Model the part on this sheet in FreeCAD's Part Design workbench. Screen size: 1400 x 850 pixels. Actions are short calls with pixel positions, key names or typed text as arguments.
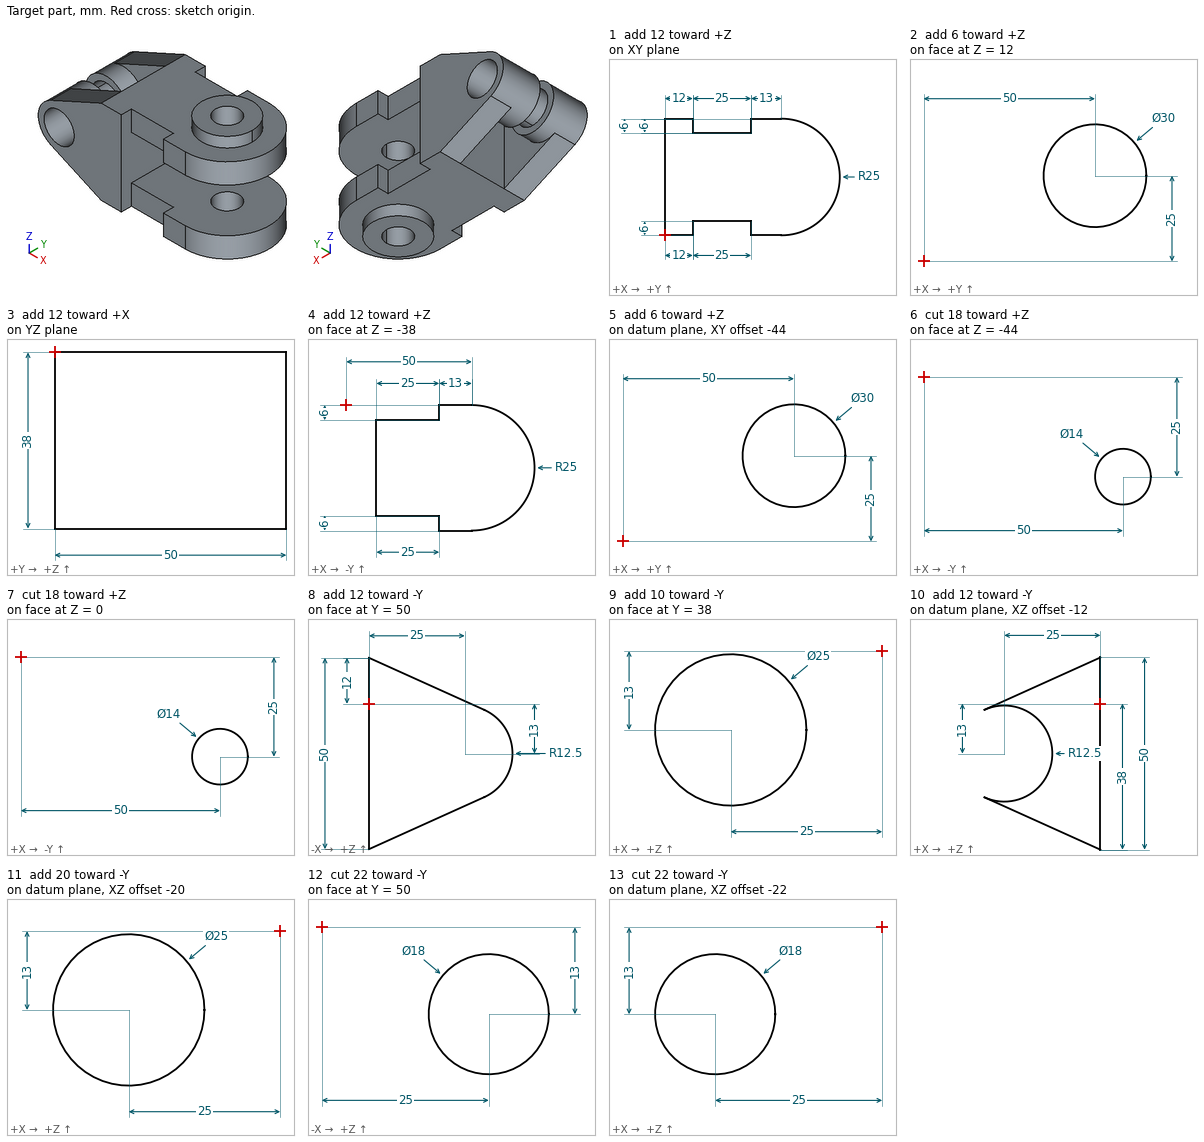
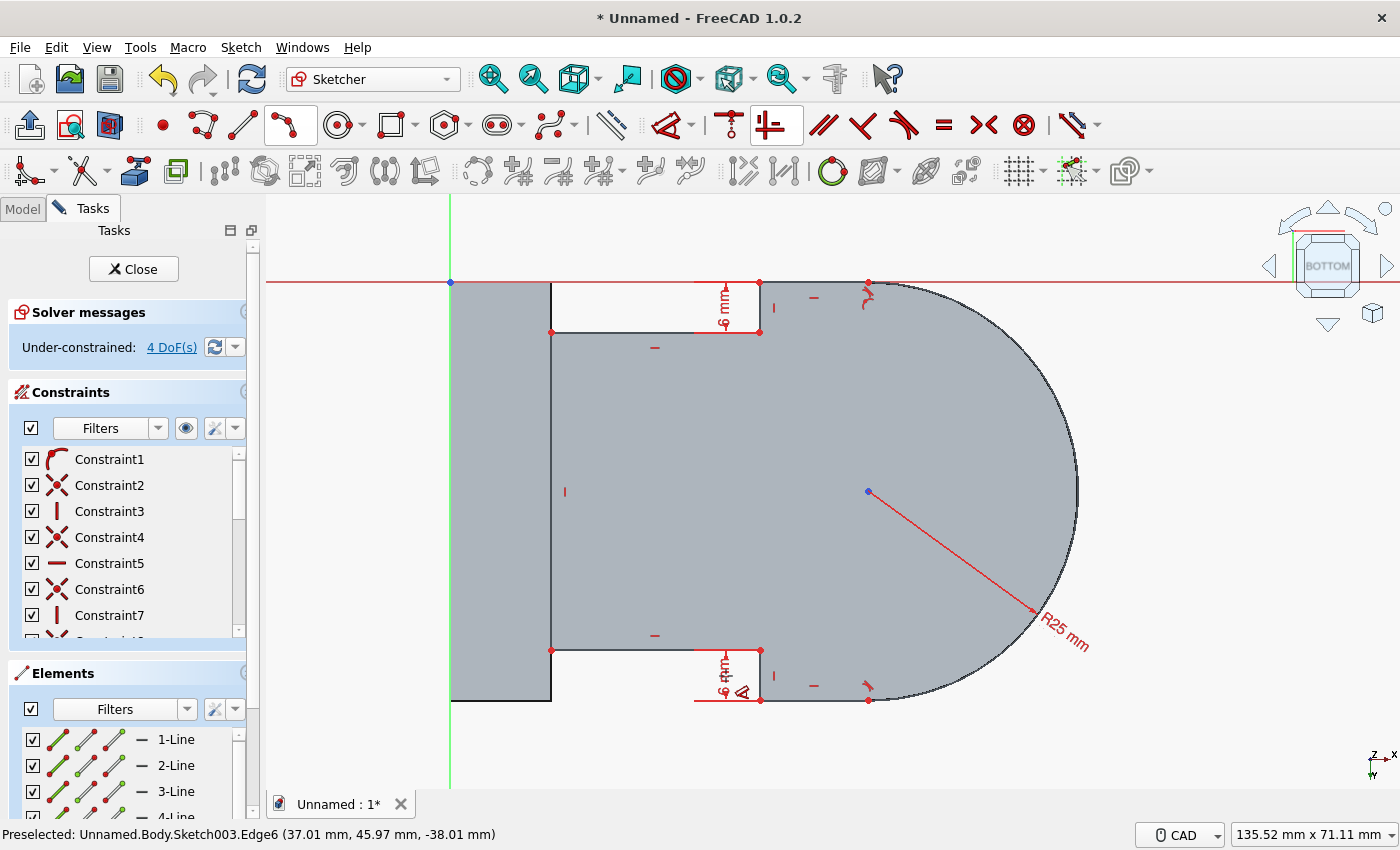
click(836, 282)
click(814, 248)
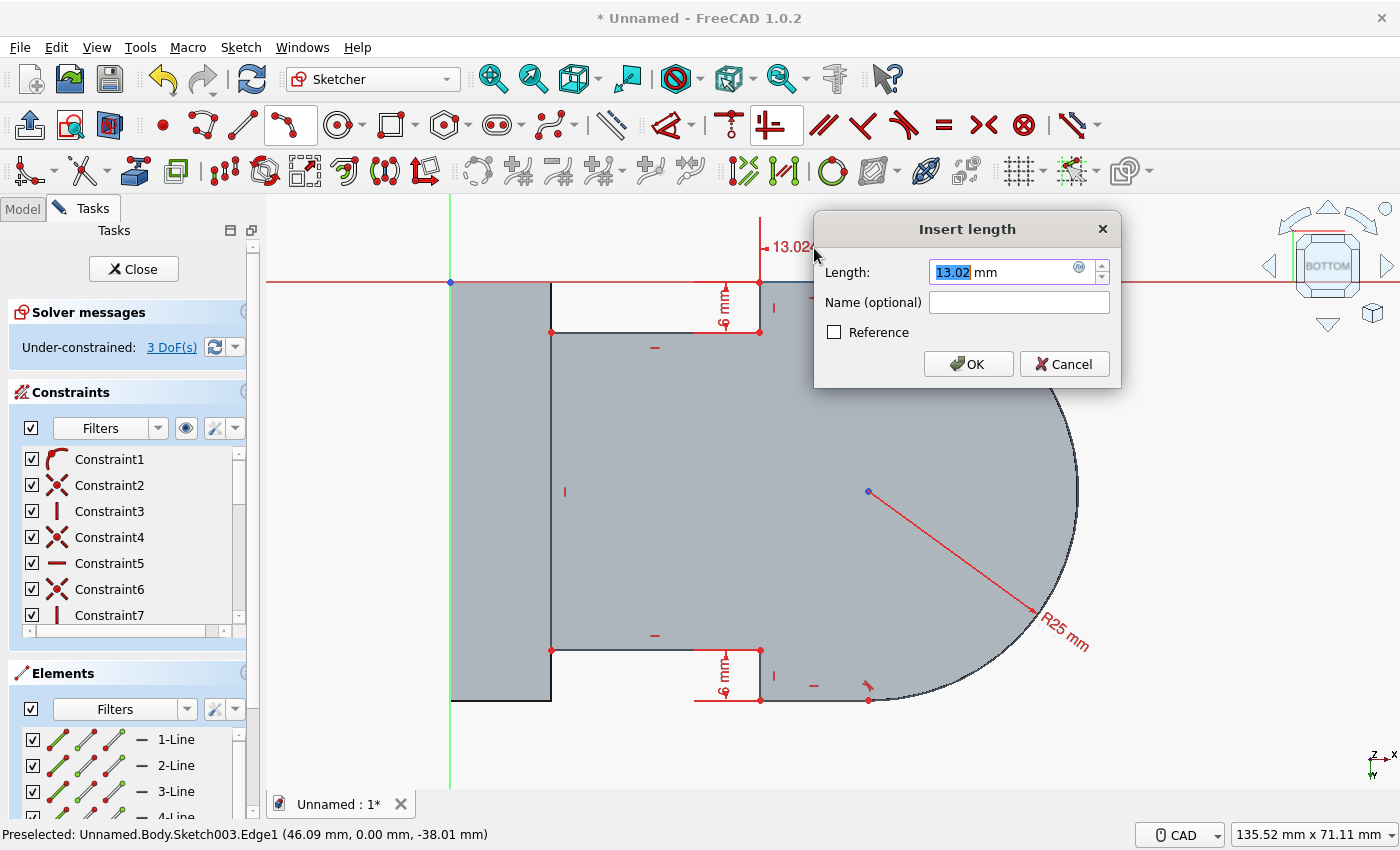
text(13)
key(Return)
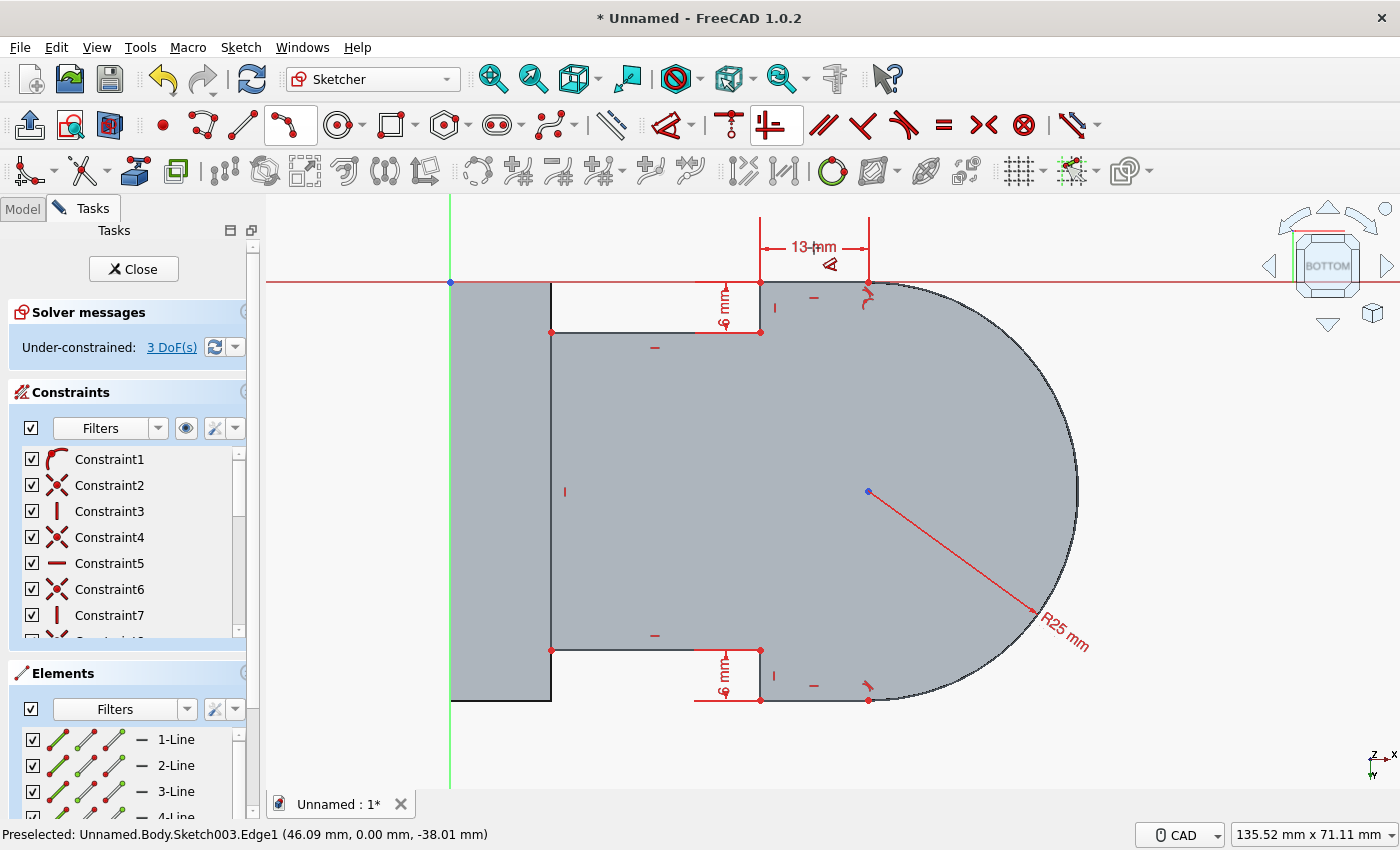
click(697, 333)
click(656, 299)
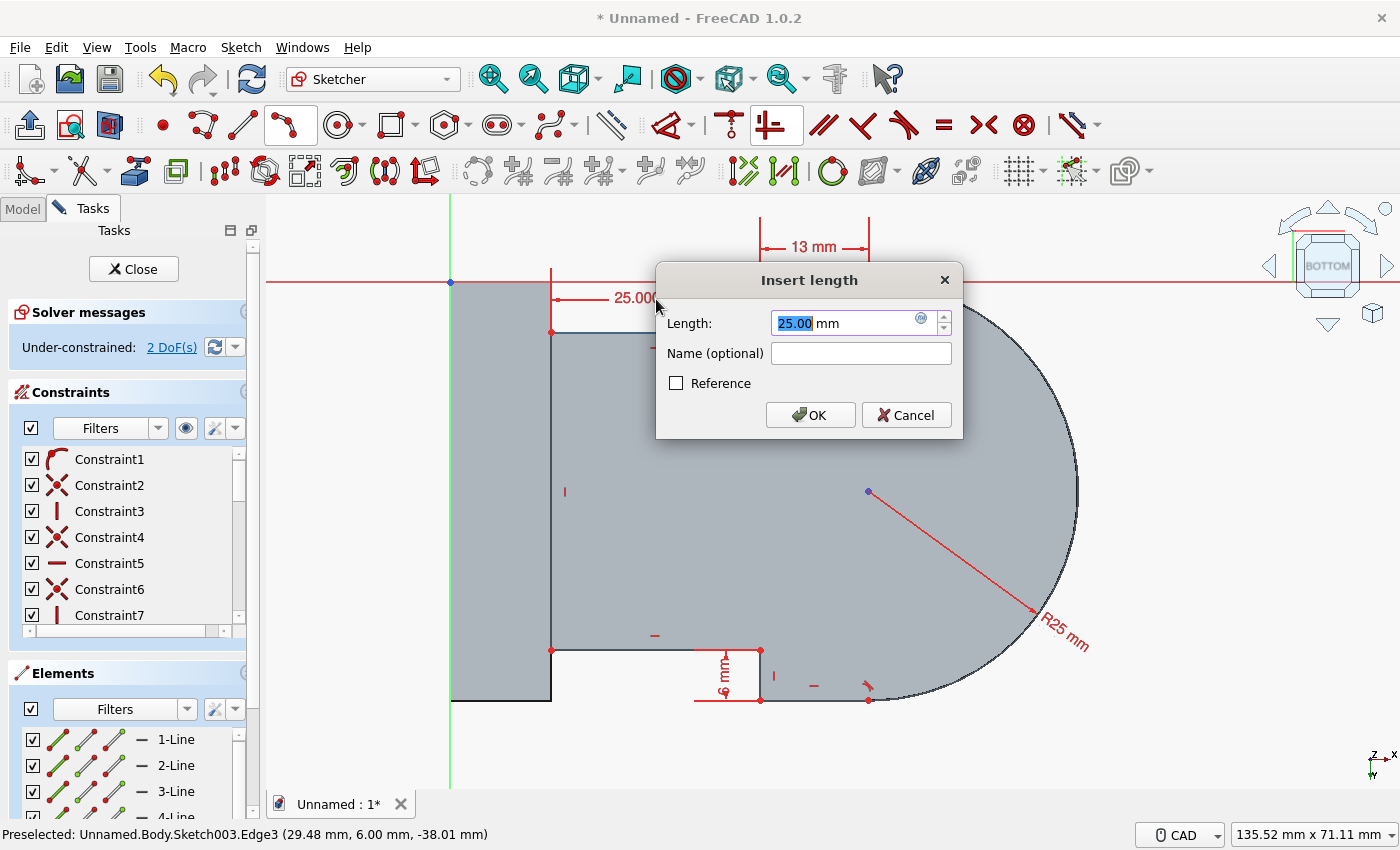
text(25)
key(Return)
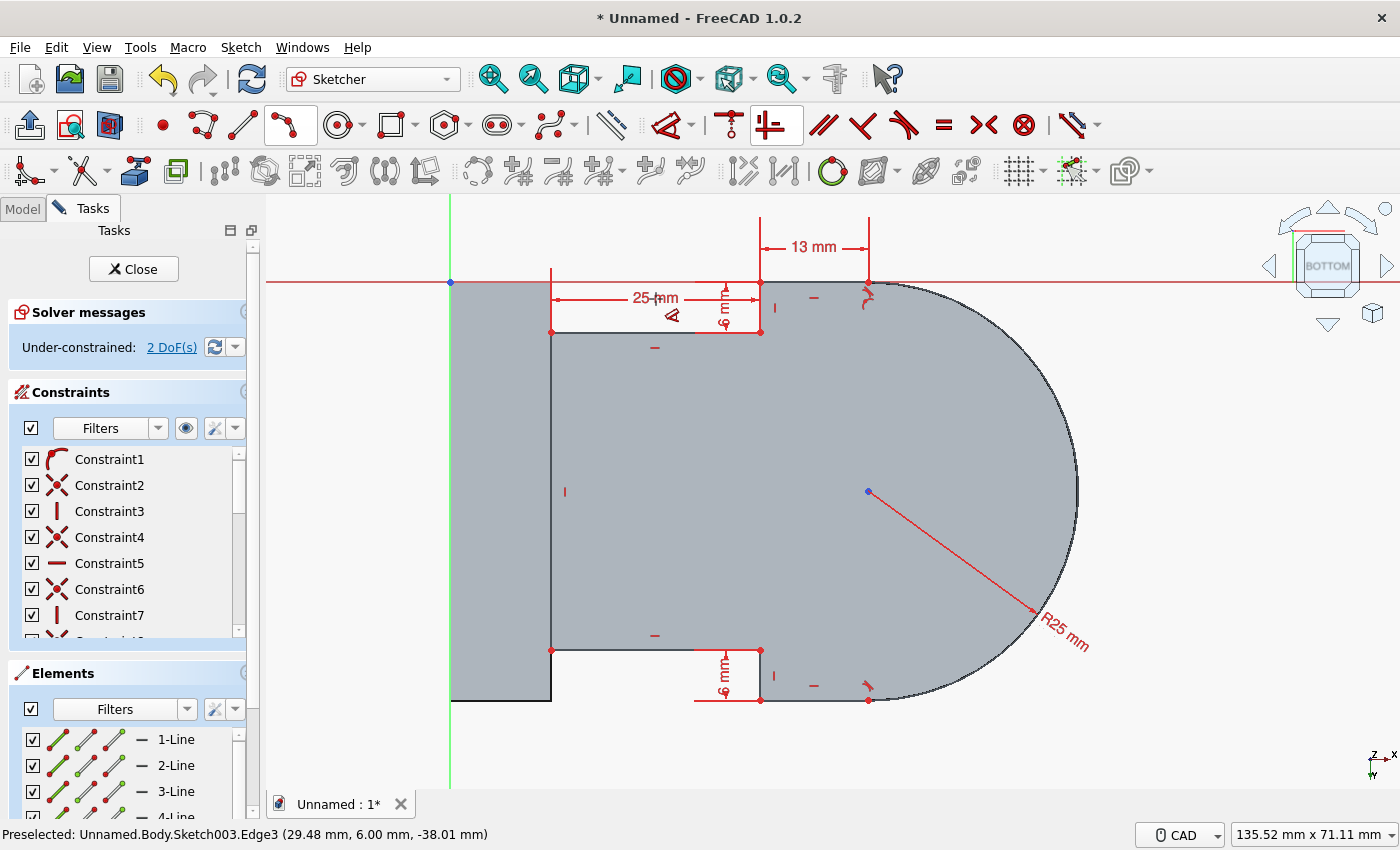
click(614, 650)
click(656, 684)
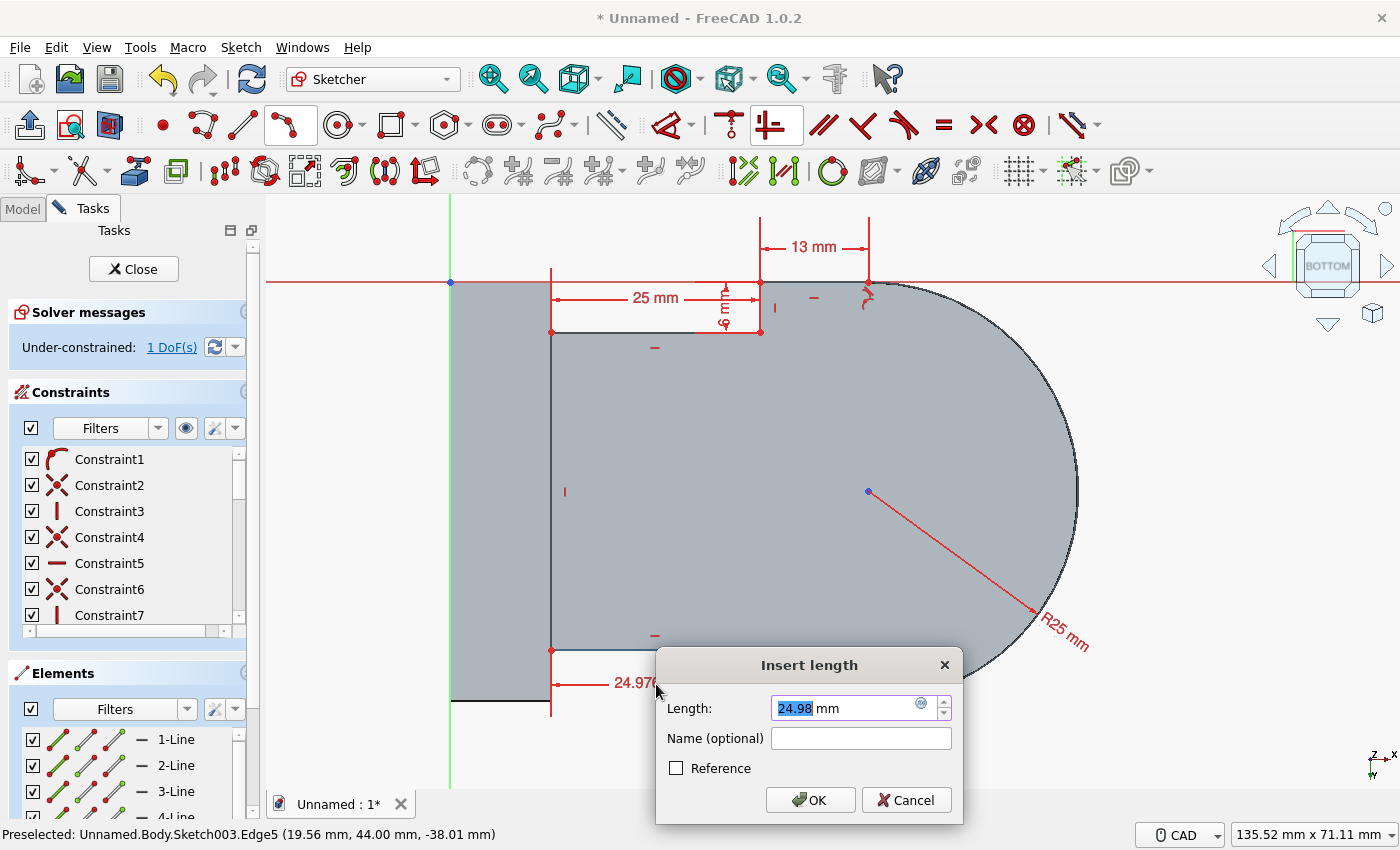
text(25)
key(Return)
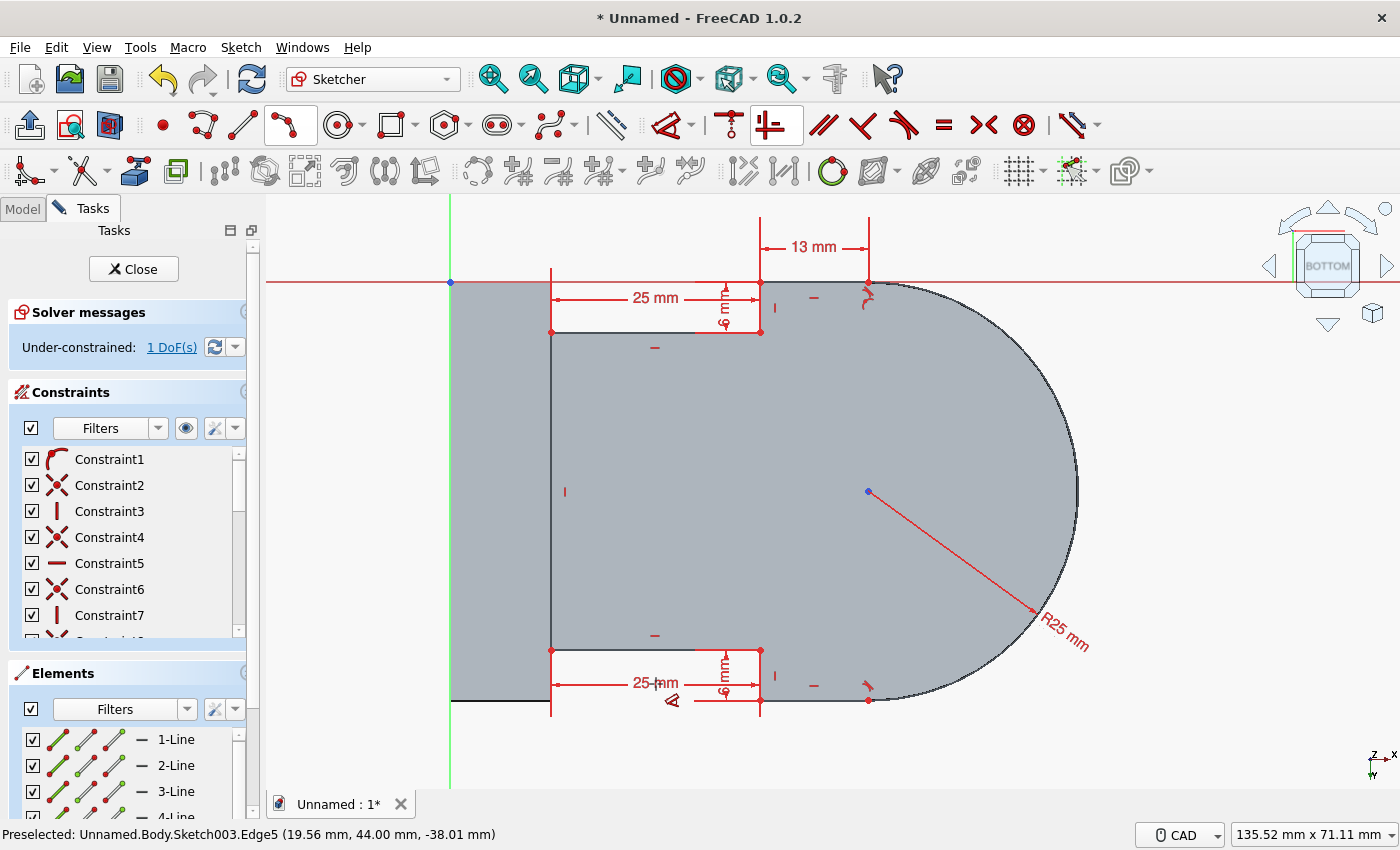
click(869, 282)
click(660, 248)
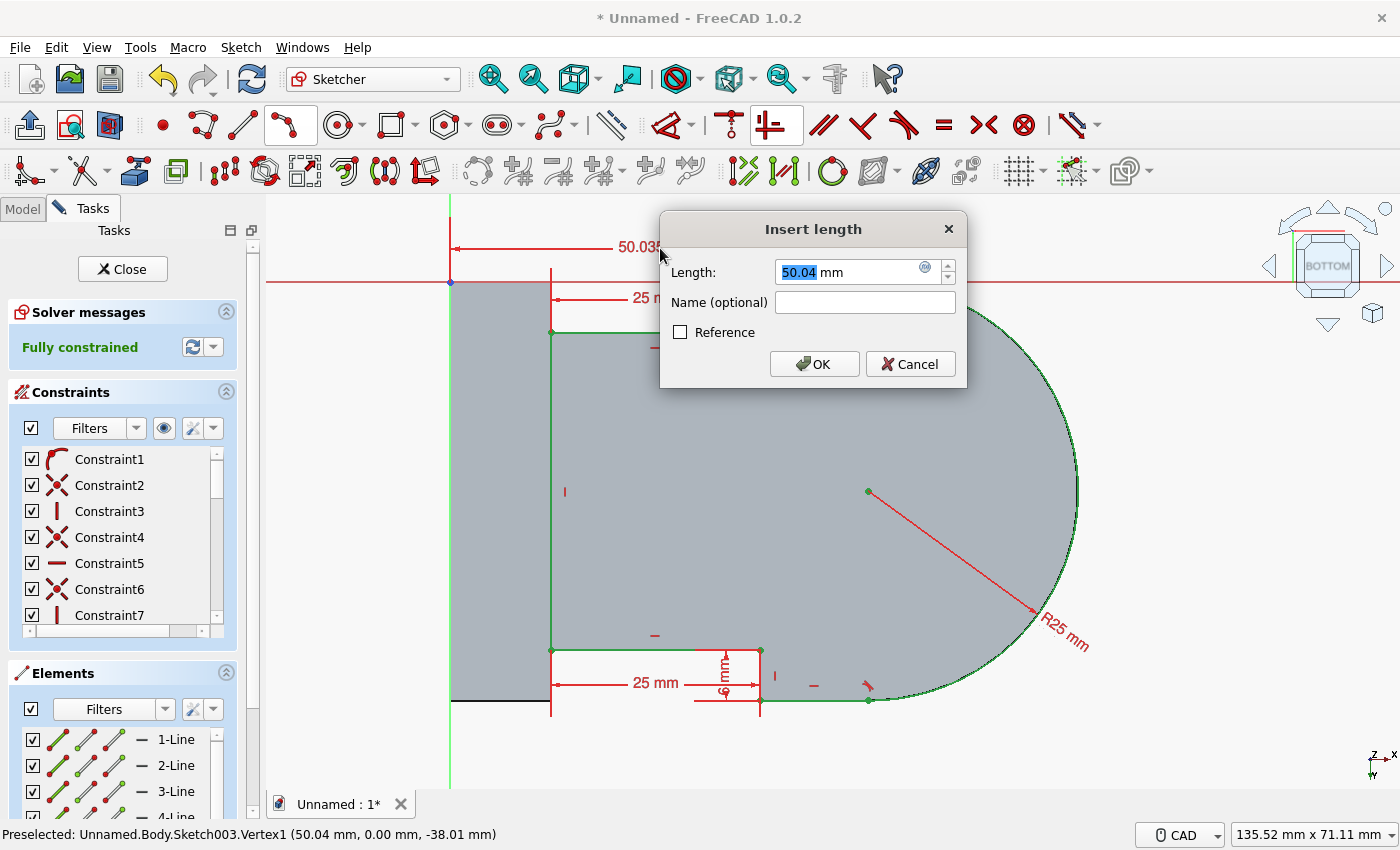
text(50)
key(Return)
key(Escape)